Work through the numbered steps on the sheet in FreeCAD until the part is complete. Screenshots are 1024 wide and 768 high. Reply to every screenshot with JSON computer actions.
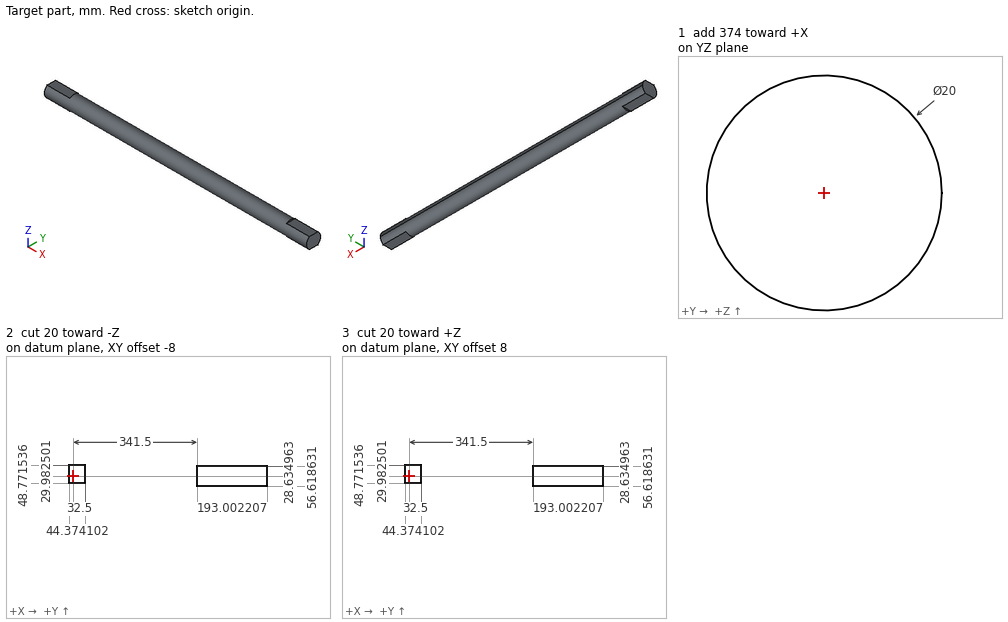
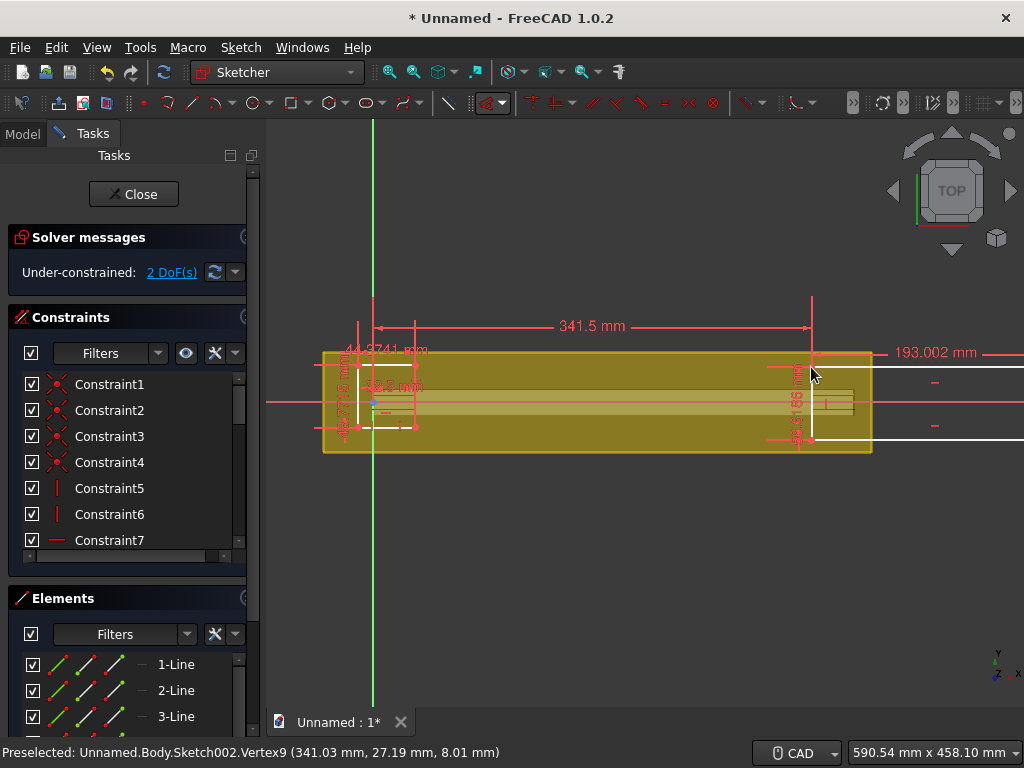
{"action": "left_click", "coordinate": [358, 365]}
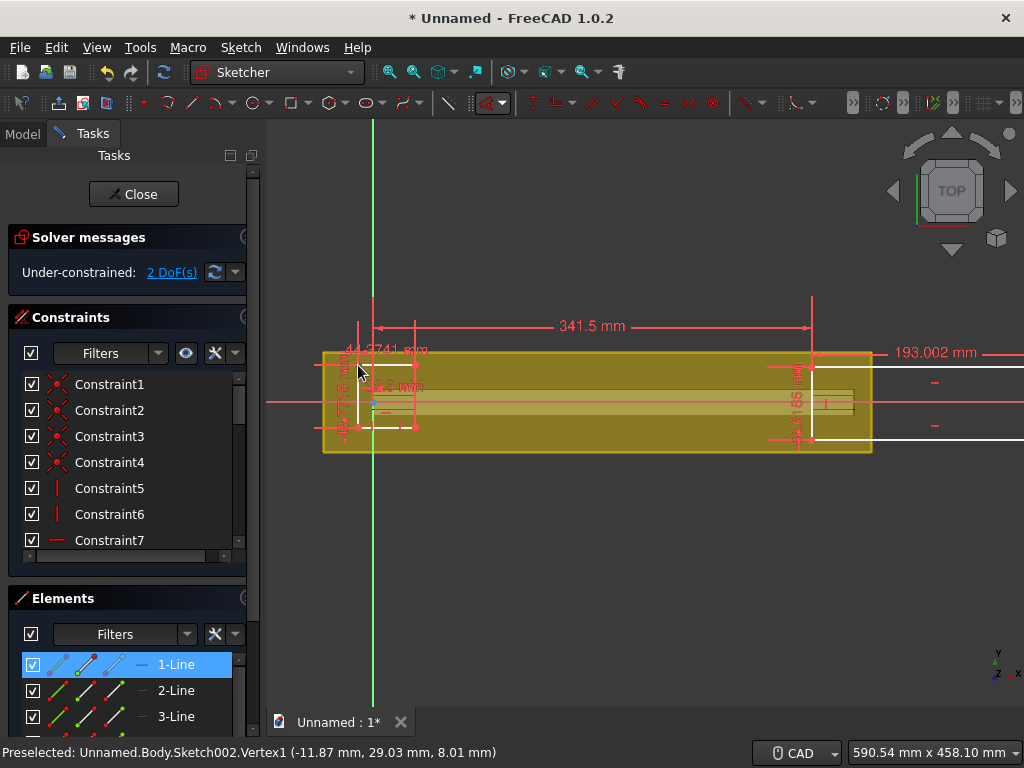
{"action": "left_click", "coordinate": [504, 104]}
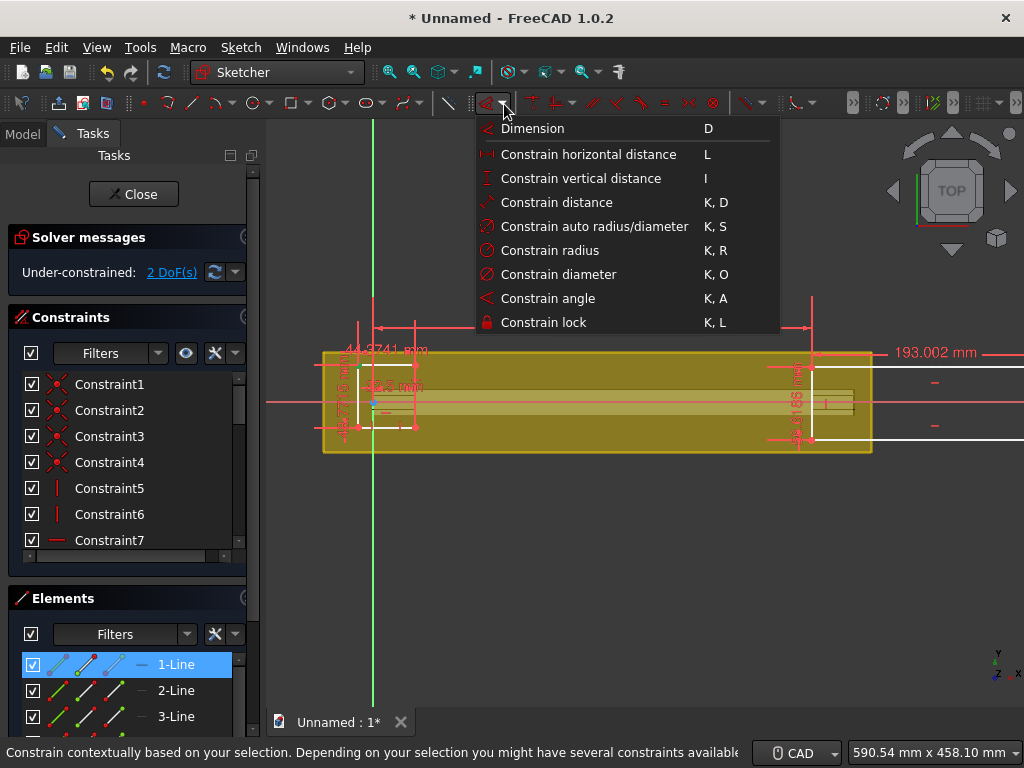
{"action": "left_click", "coordinate": [628, 178]}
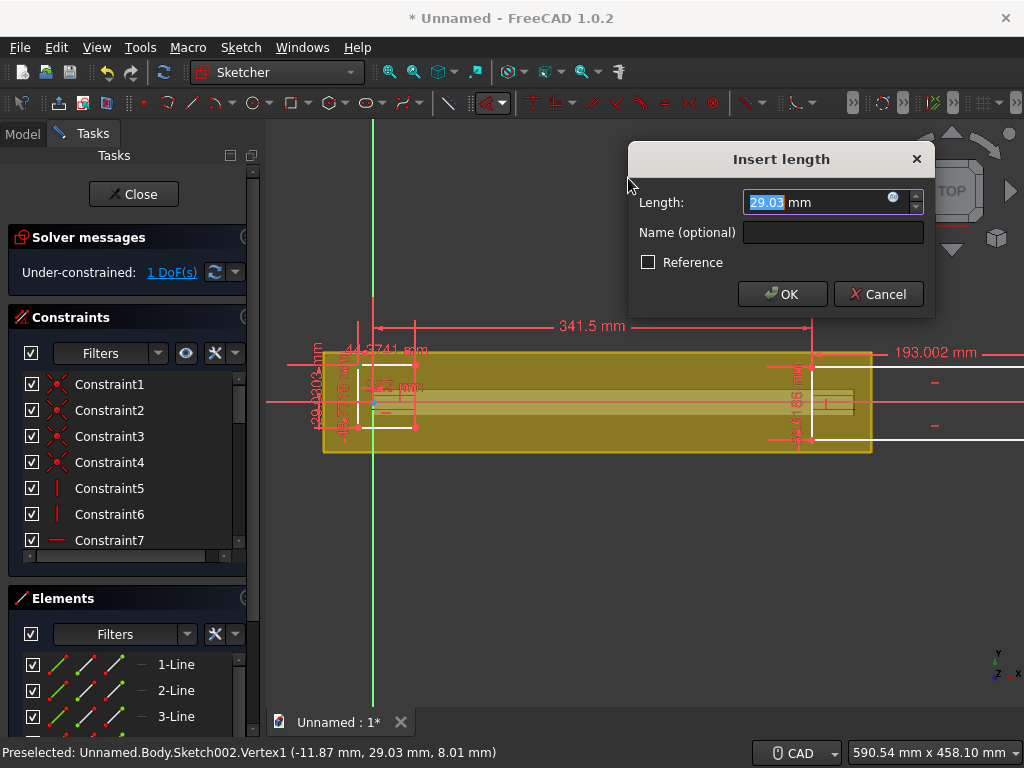
{"action": "type", "text": "29.982501"}
{"action": "key", "text": "Return"}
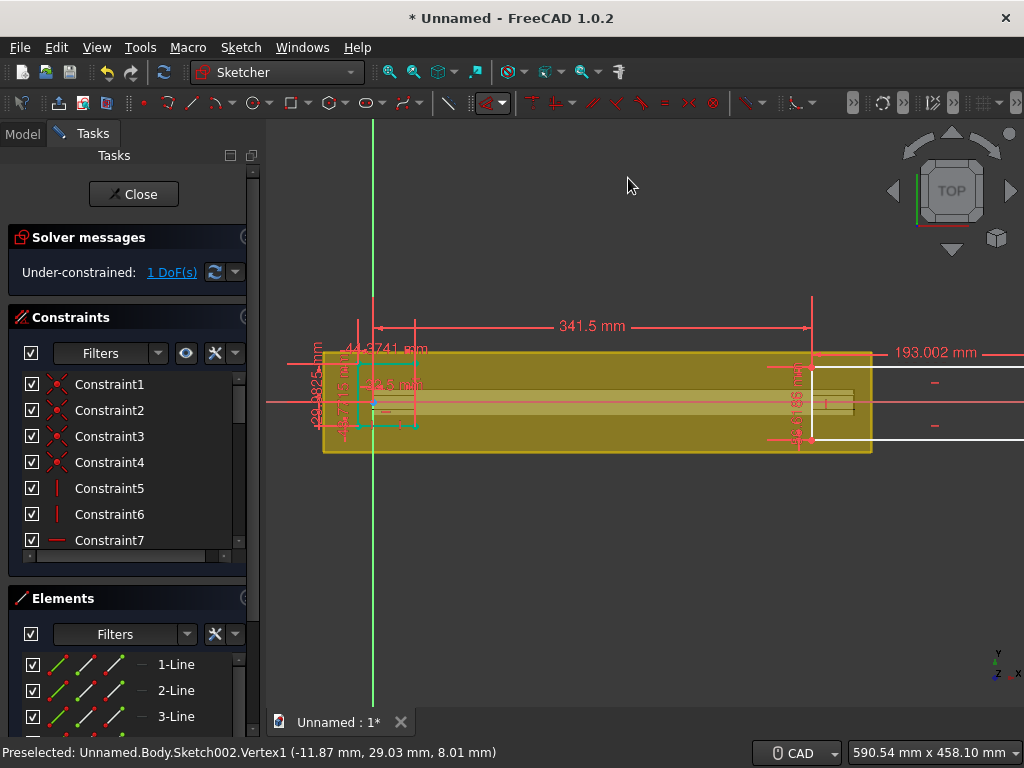
{"action": "left_click", "coordinate": [812, 367]}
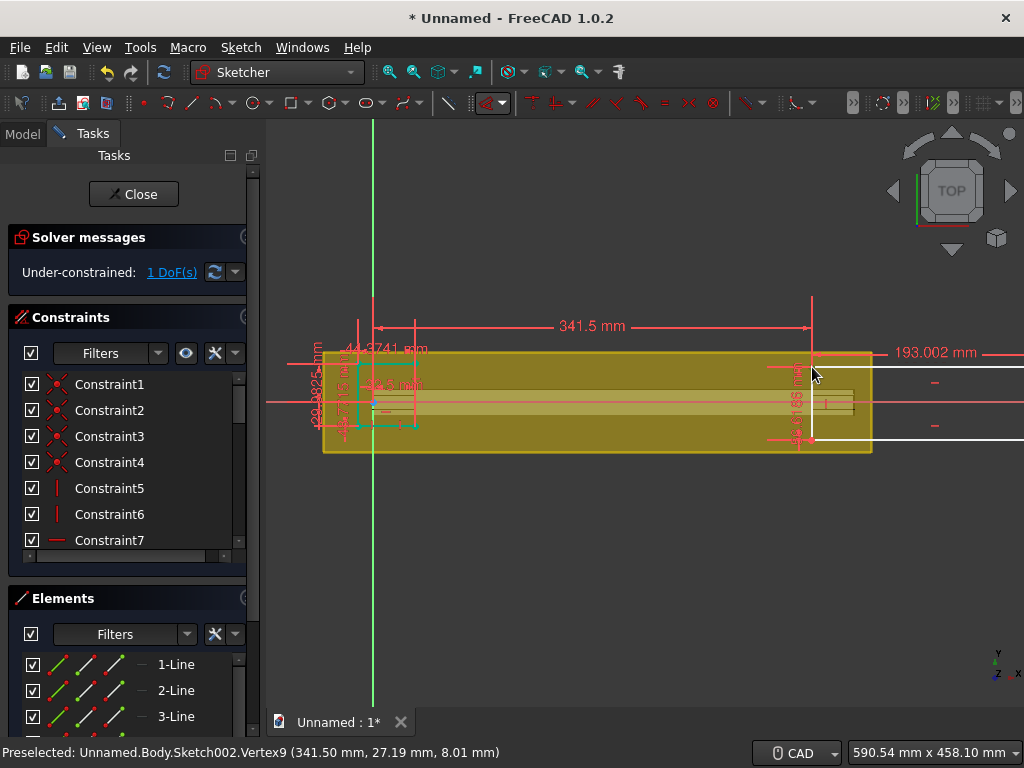
{"action": "left_click", "coordinate": [504, 104]}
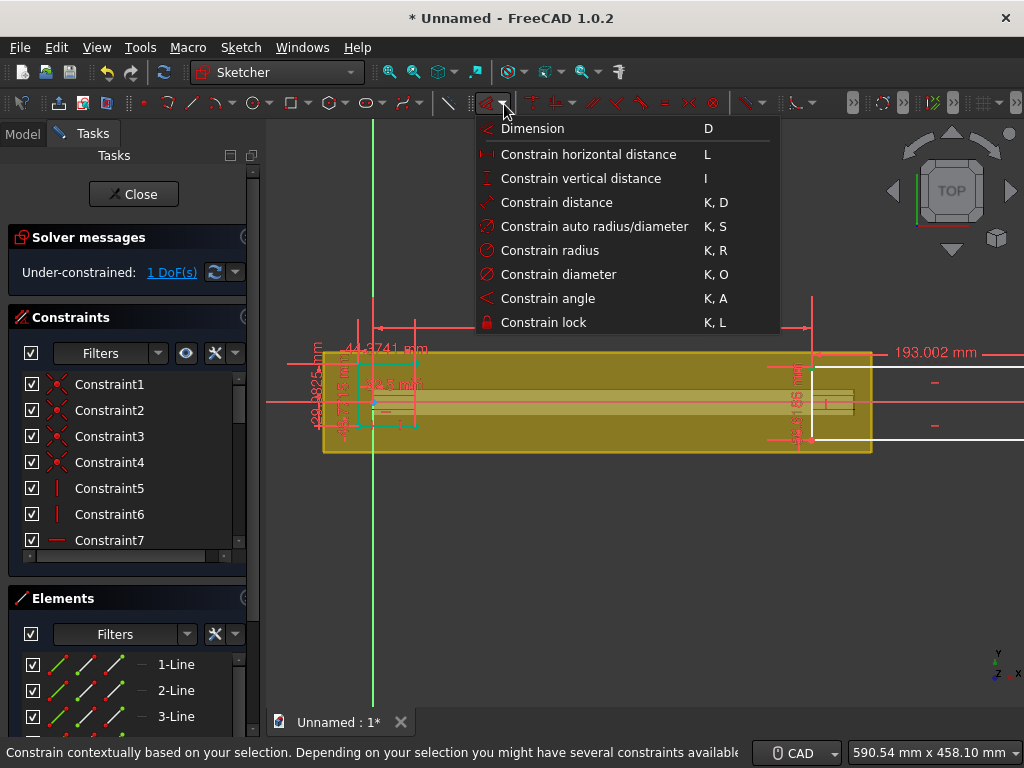
{"action": "left_click", "coordinate": [628, 178]}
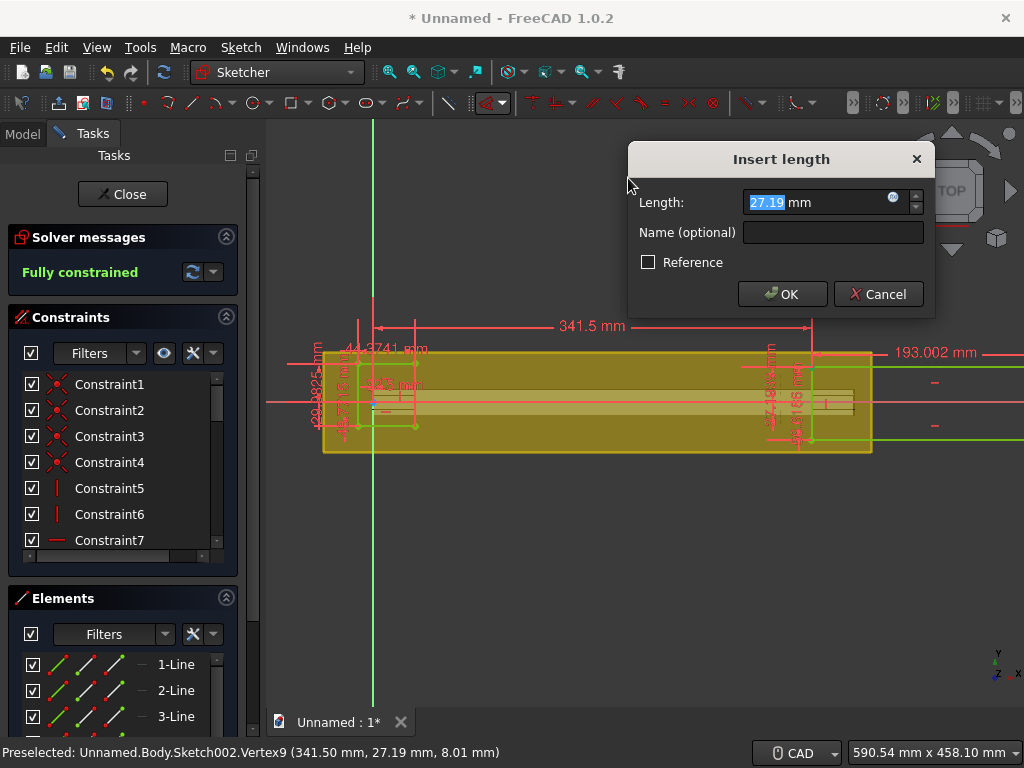
{"action": "type", "text": "28.634963"}
{"action": "key", "text": "Return"}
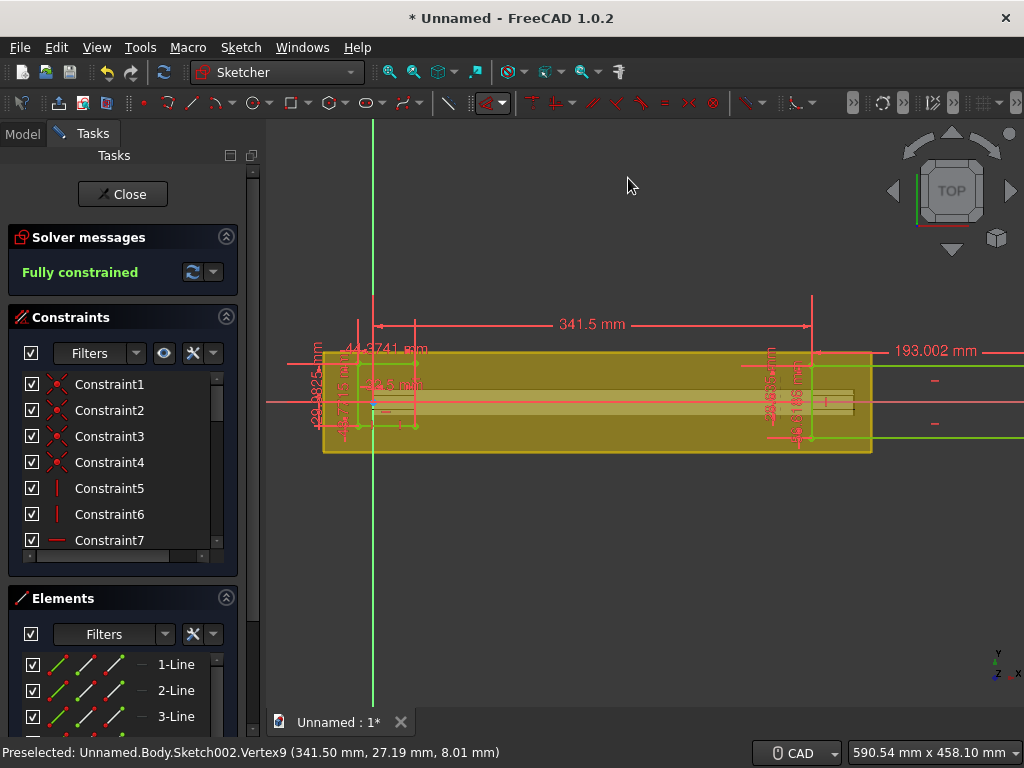
{"action": "left_click", "coordinate": [123, 194]}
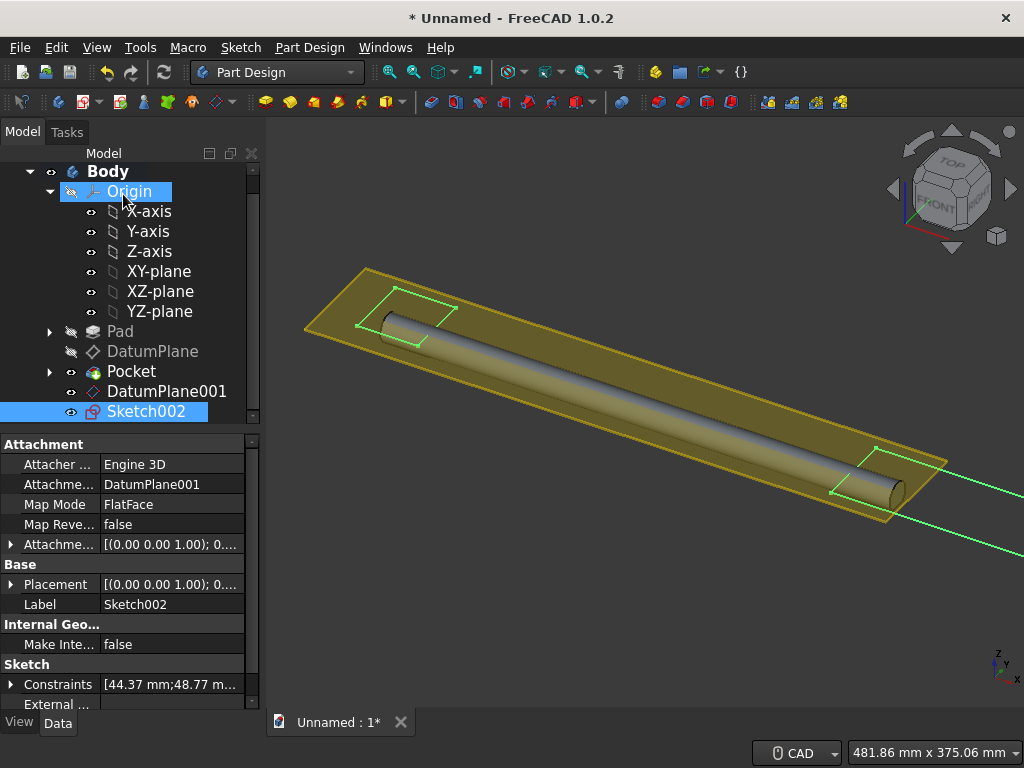
{"action": "left_click", "coordinate": [432, 102]}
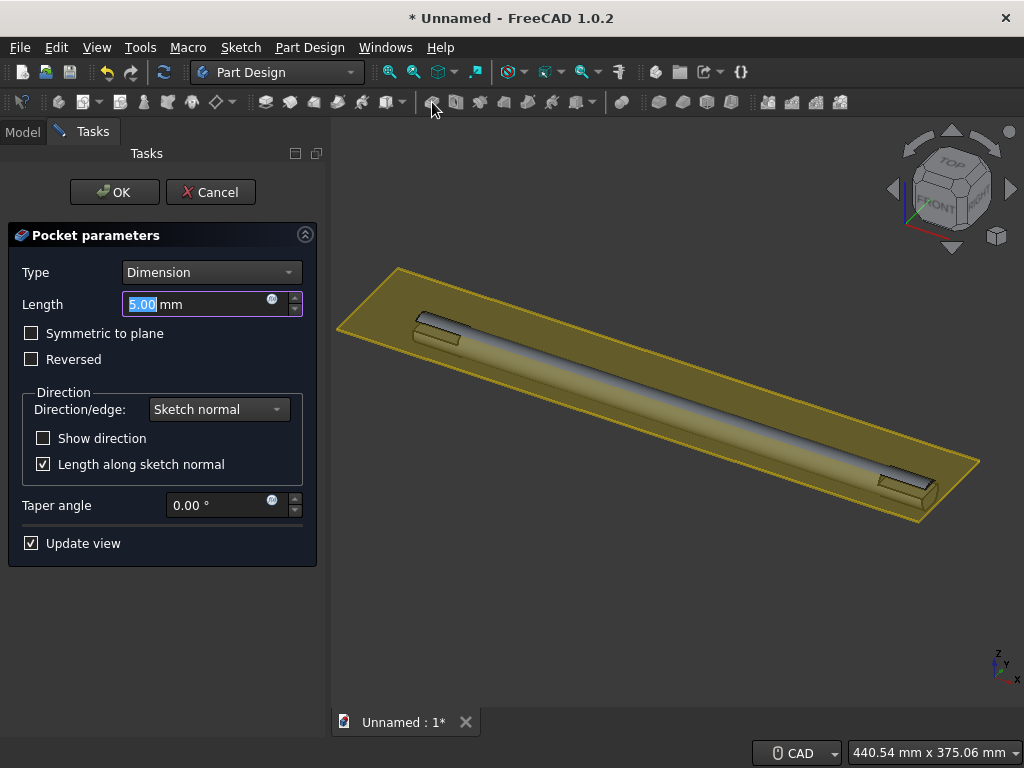
{"action": "type", "text": "20"}
{"action": "key", "text": "Tab"}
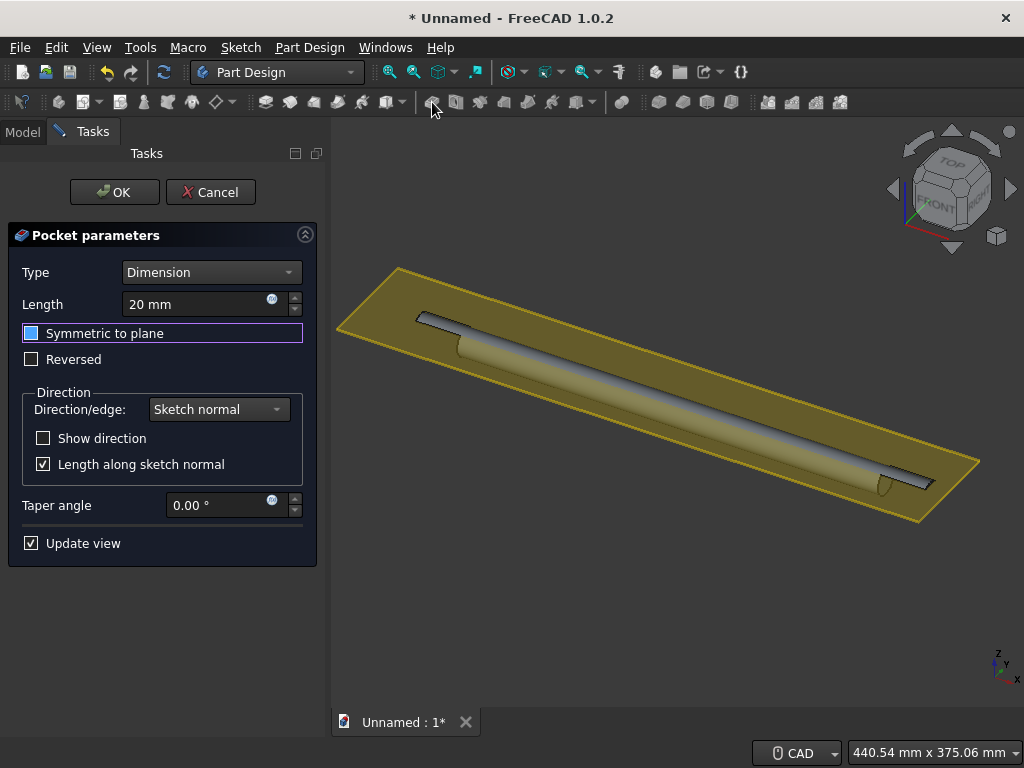
{"action": "left_click", "coordinate": [30, 359]}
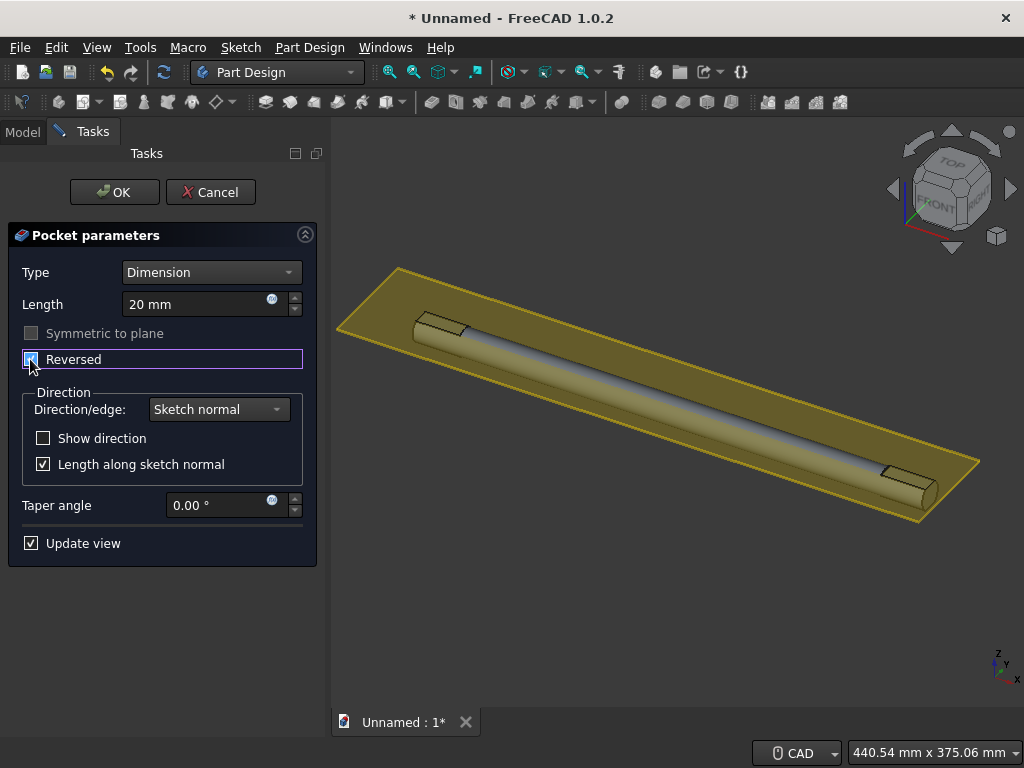
{"action": "left_click", "coordinate": [115, 192]}